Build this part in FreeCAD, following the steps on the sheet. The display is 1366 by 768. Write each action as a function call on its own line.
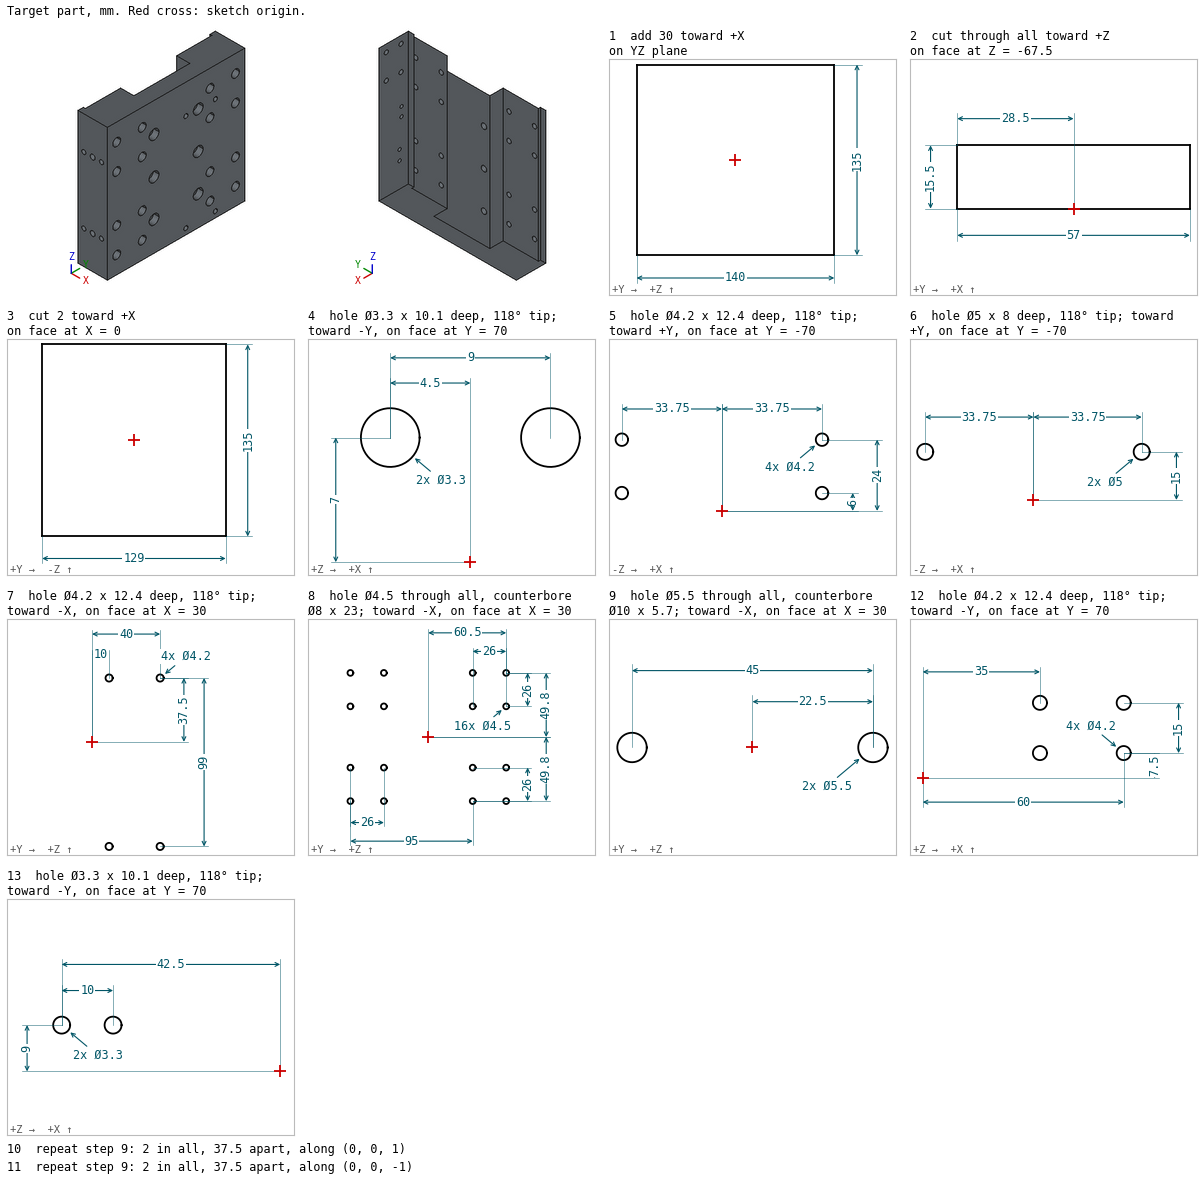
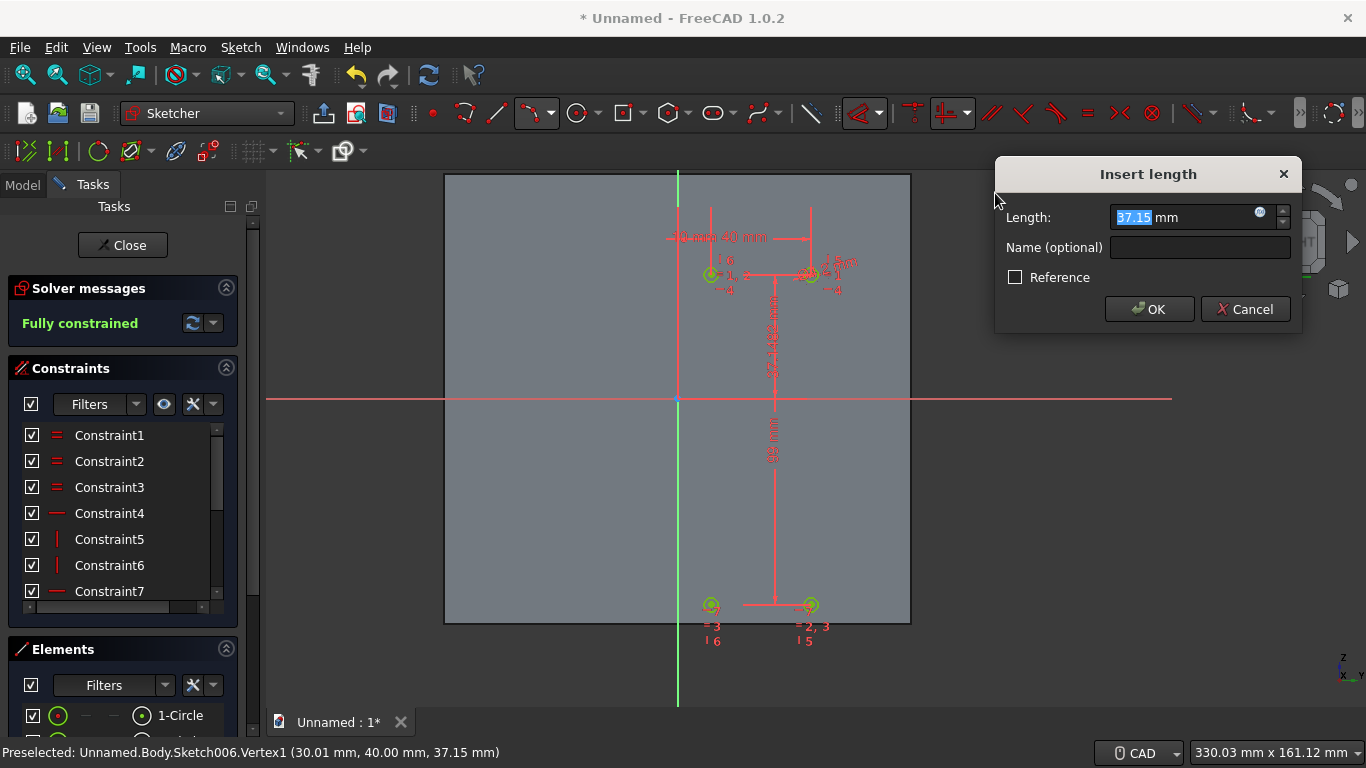
text(37.5)
key(Return)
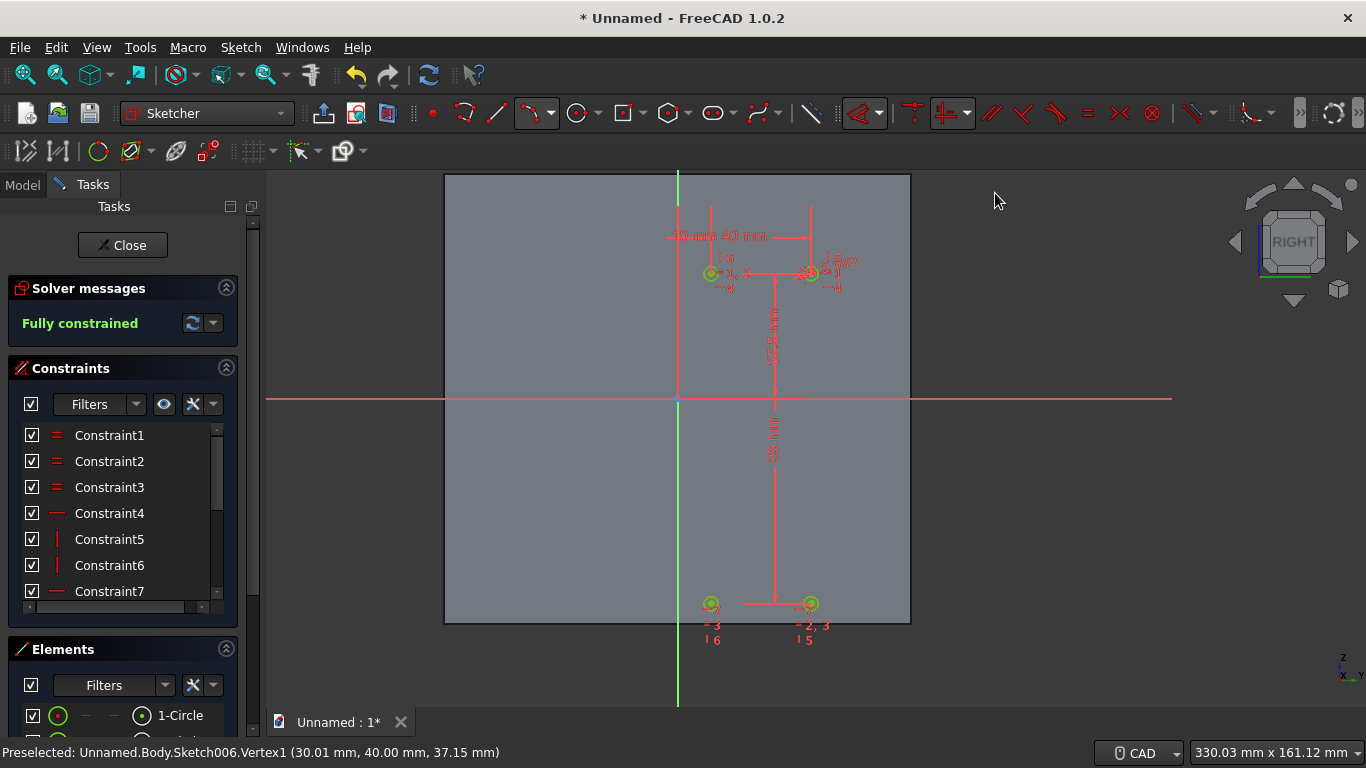
click(123, 245)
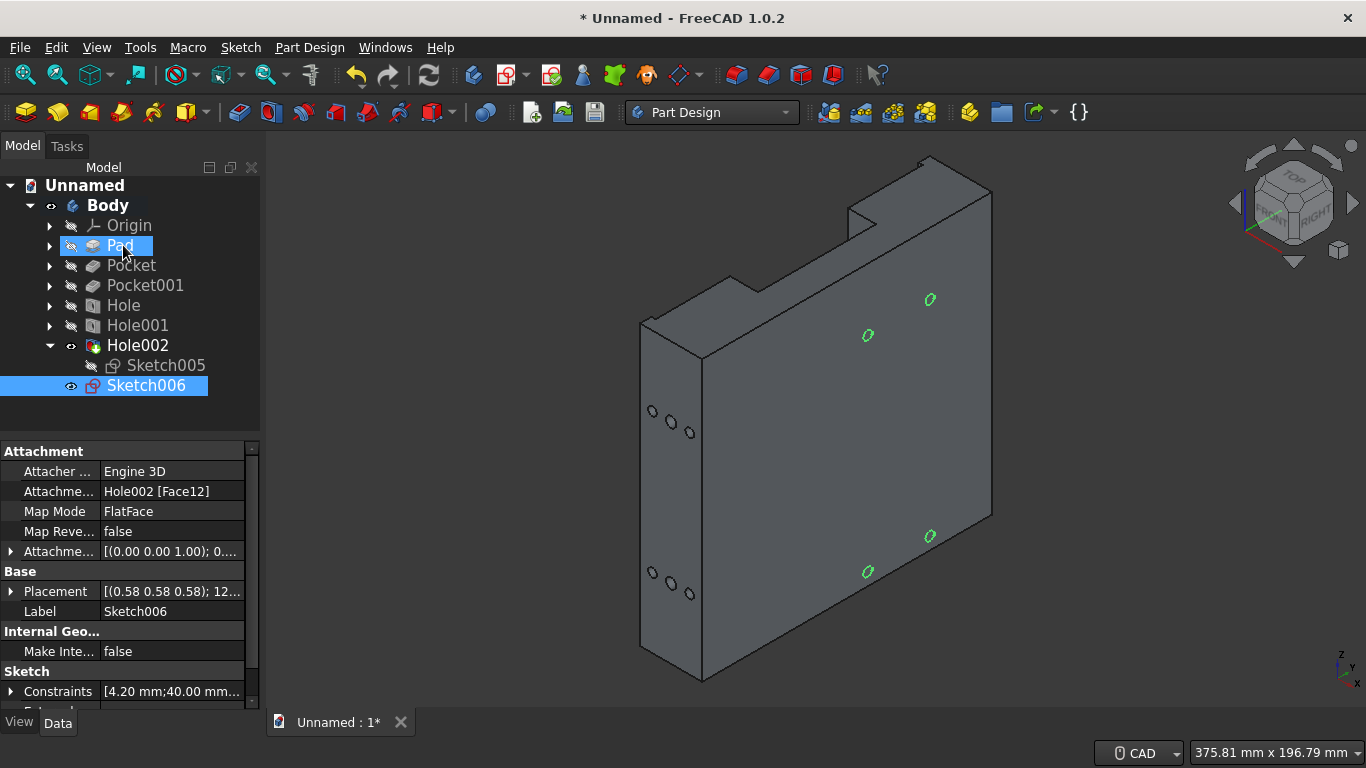
click(272, 112)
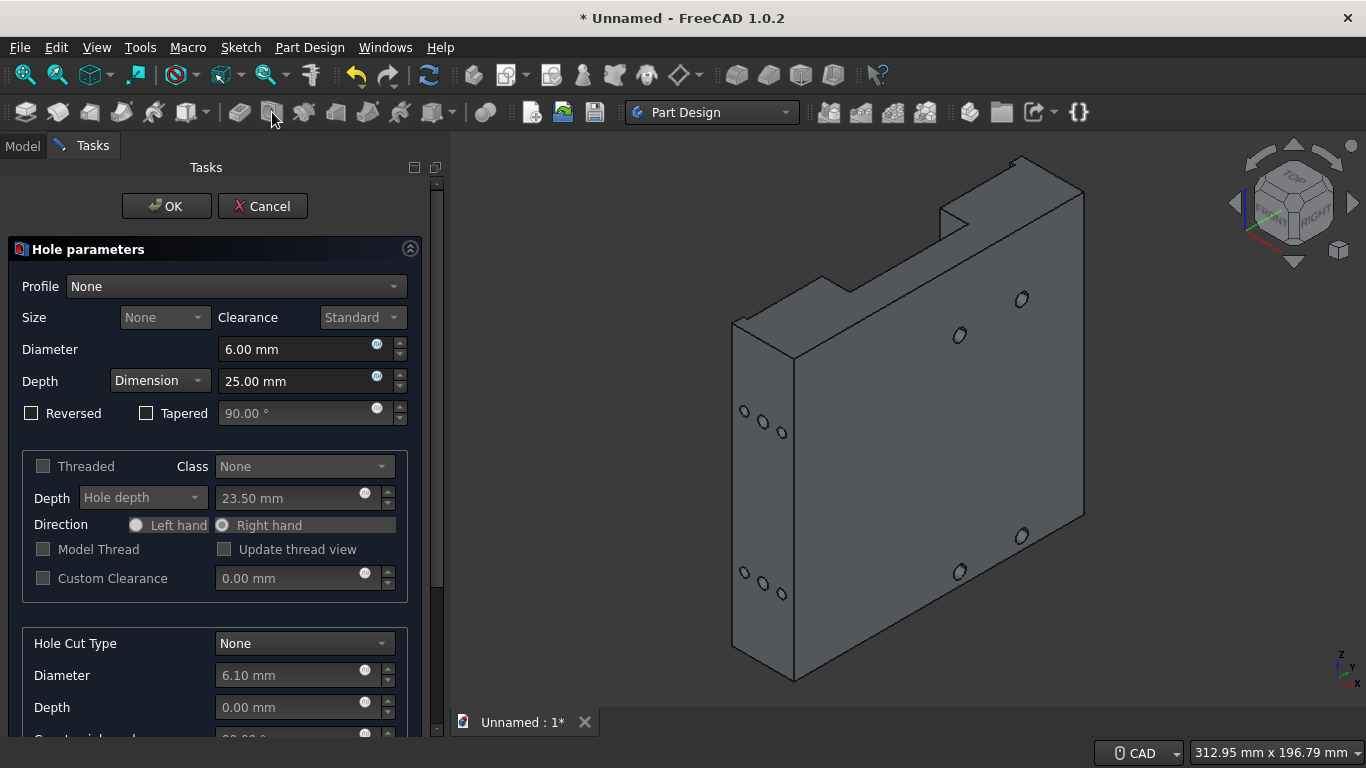
triple_click(305, 349)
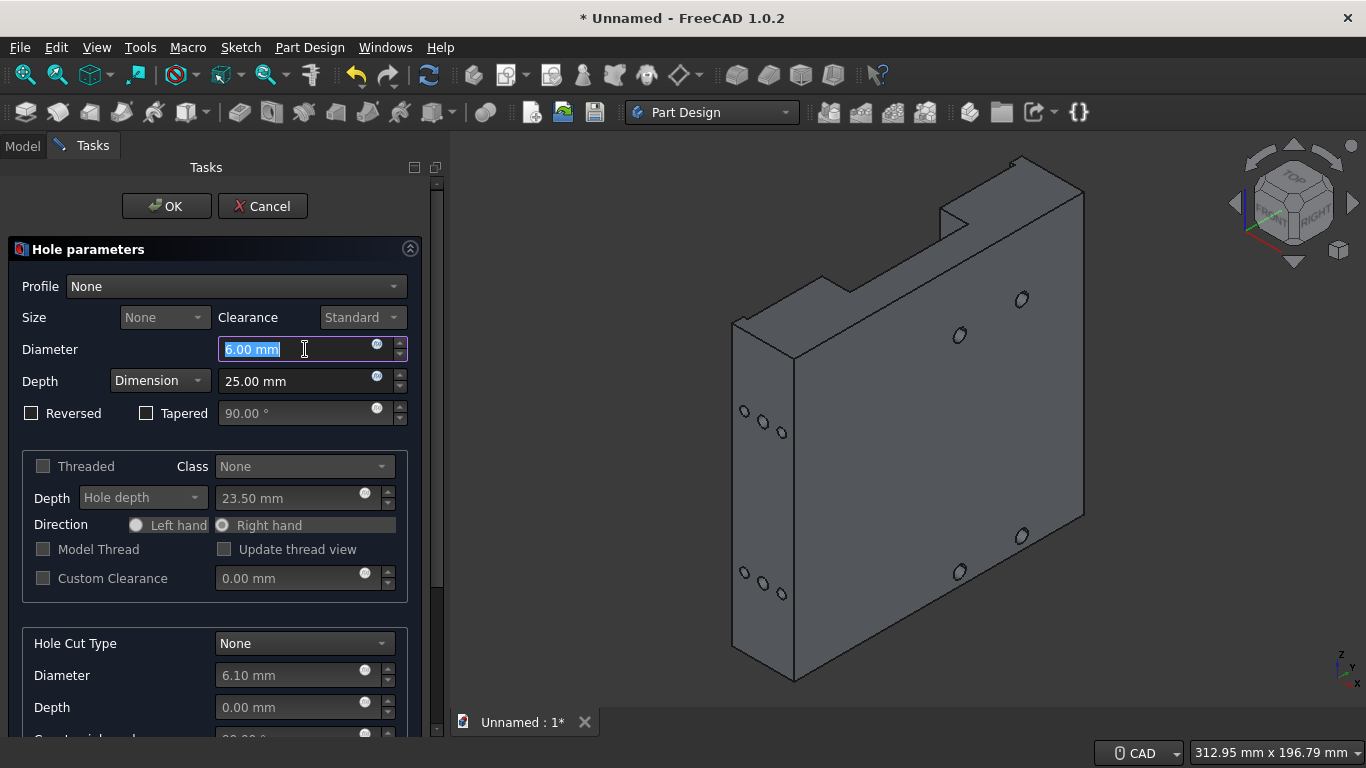
text(4.2)
key(Tab)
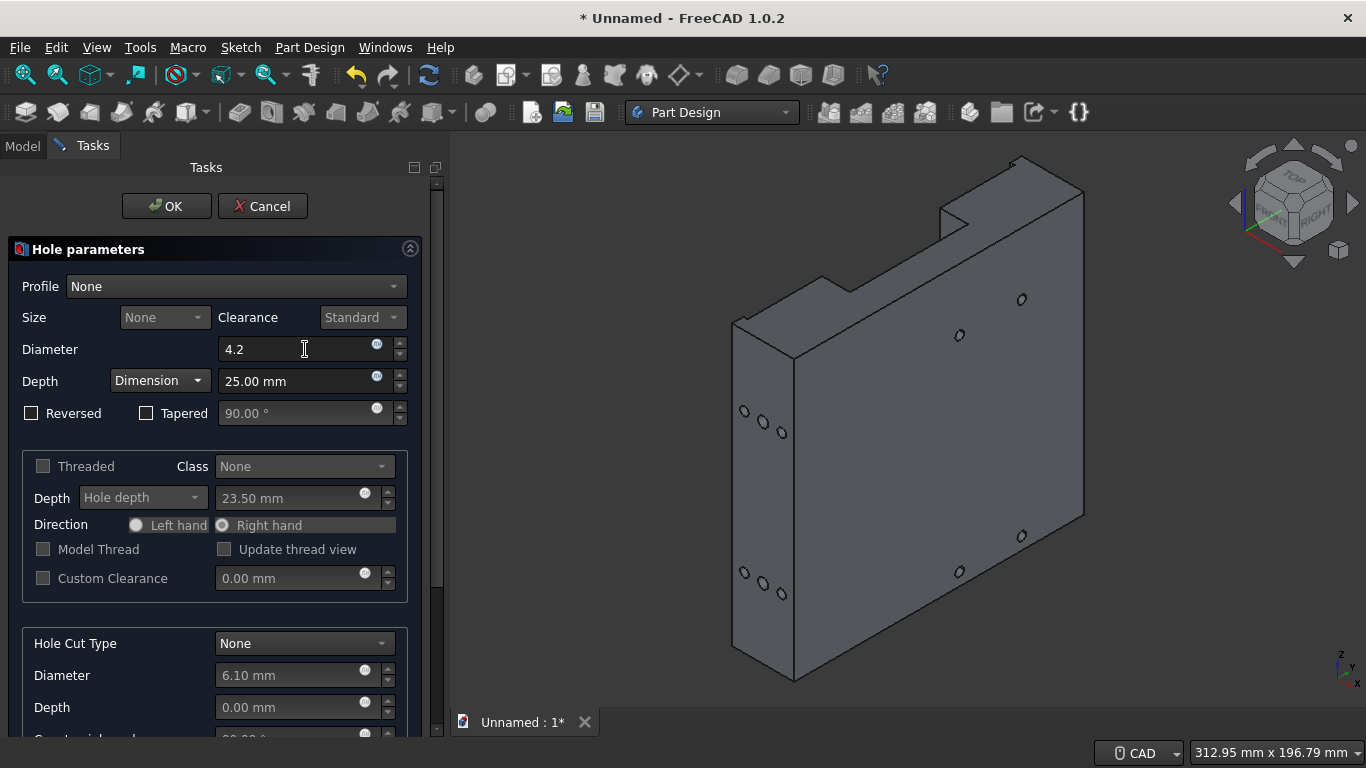
triple_click(305, 381)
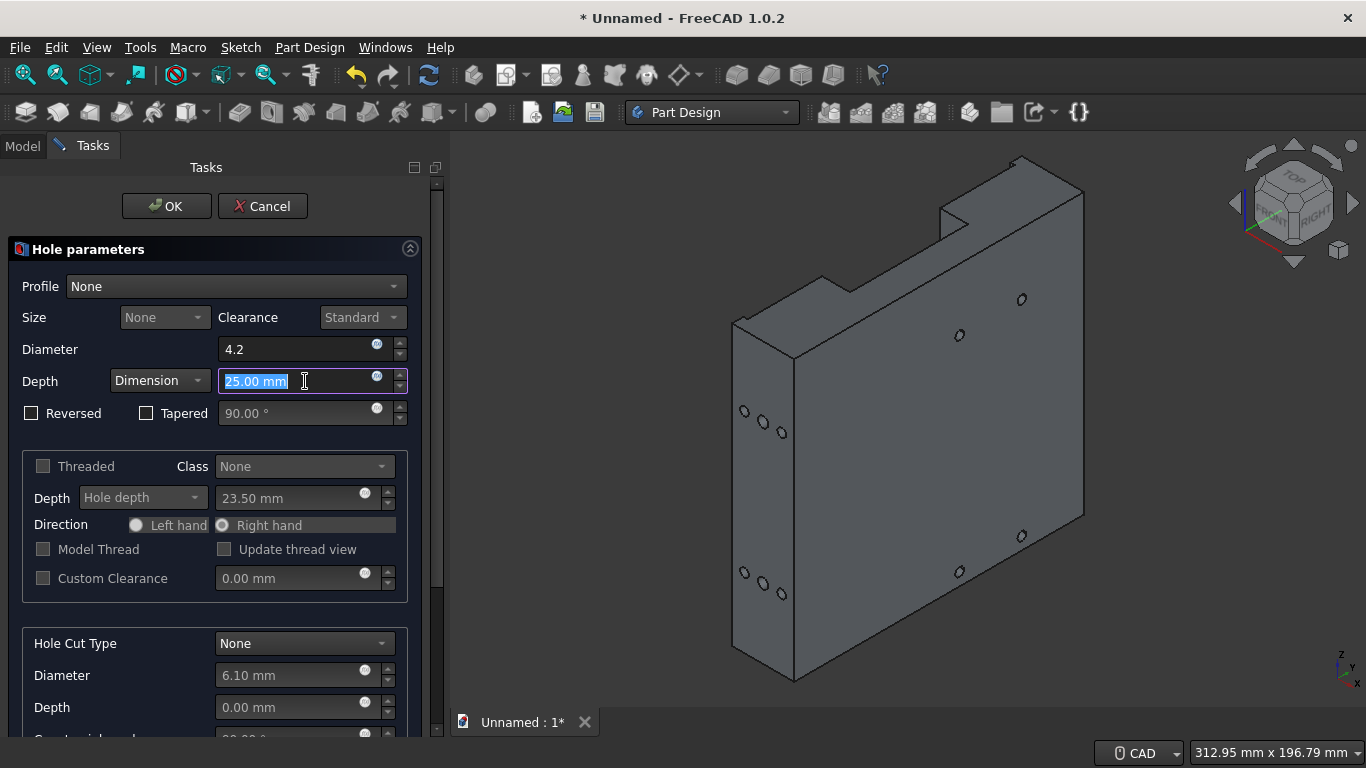
text(12.4)
key(Tab)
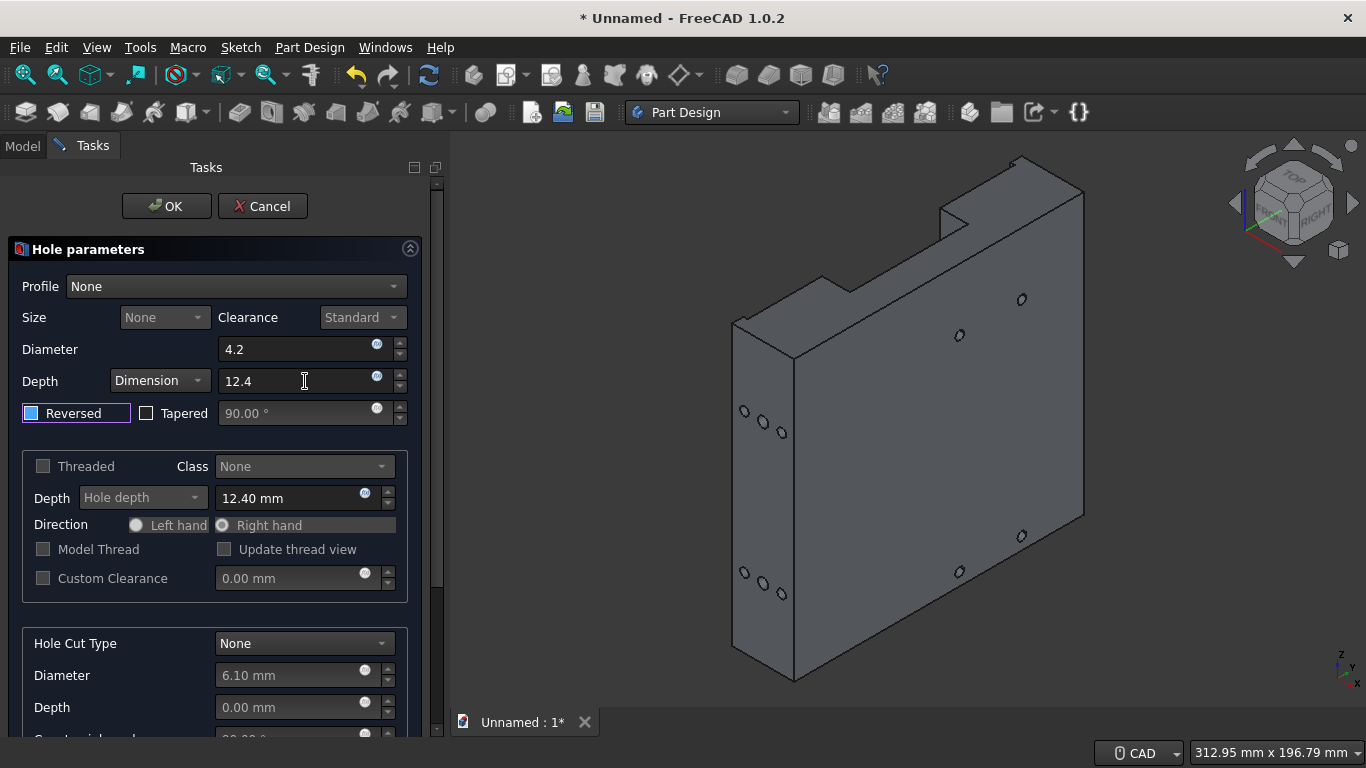
click(167, 206)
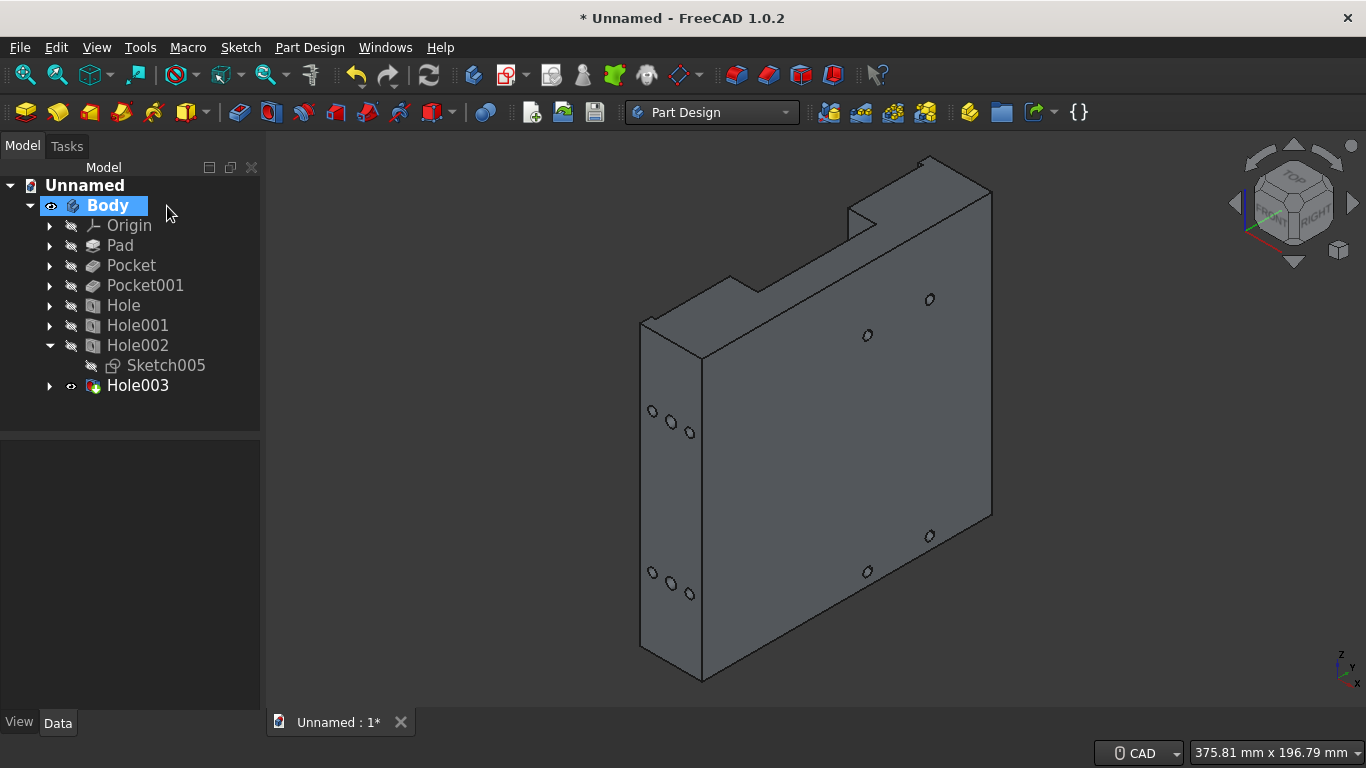
click(806, 506)